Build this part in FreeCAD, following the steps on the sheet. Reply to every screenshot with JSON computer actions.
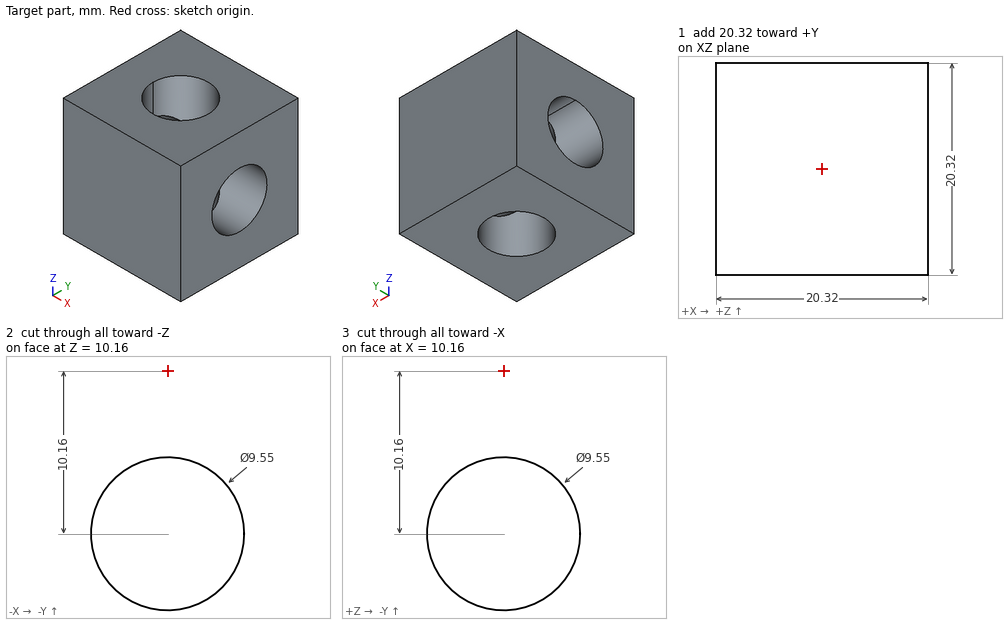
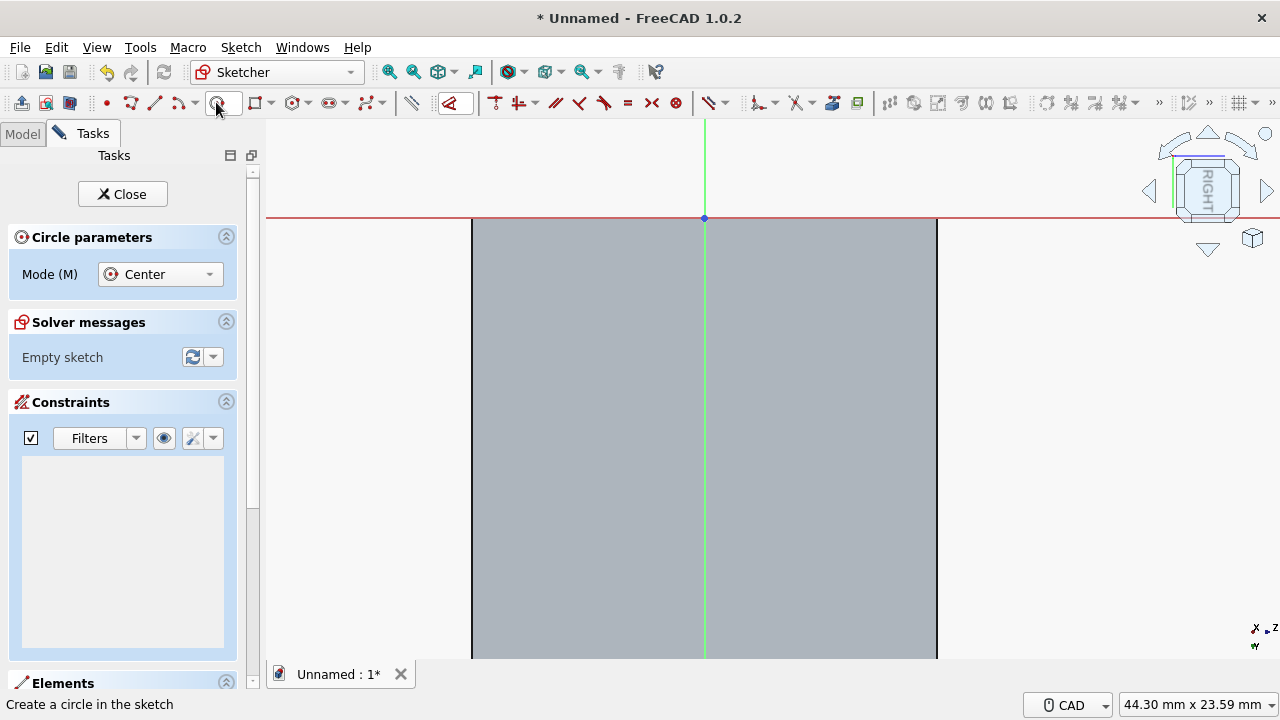
{"action": "left_click", "coordinate": [705, 451]}
{"action": "mouse_move", "coordinate": [782, 373]}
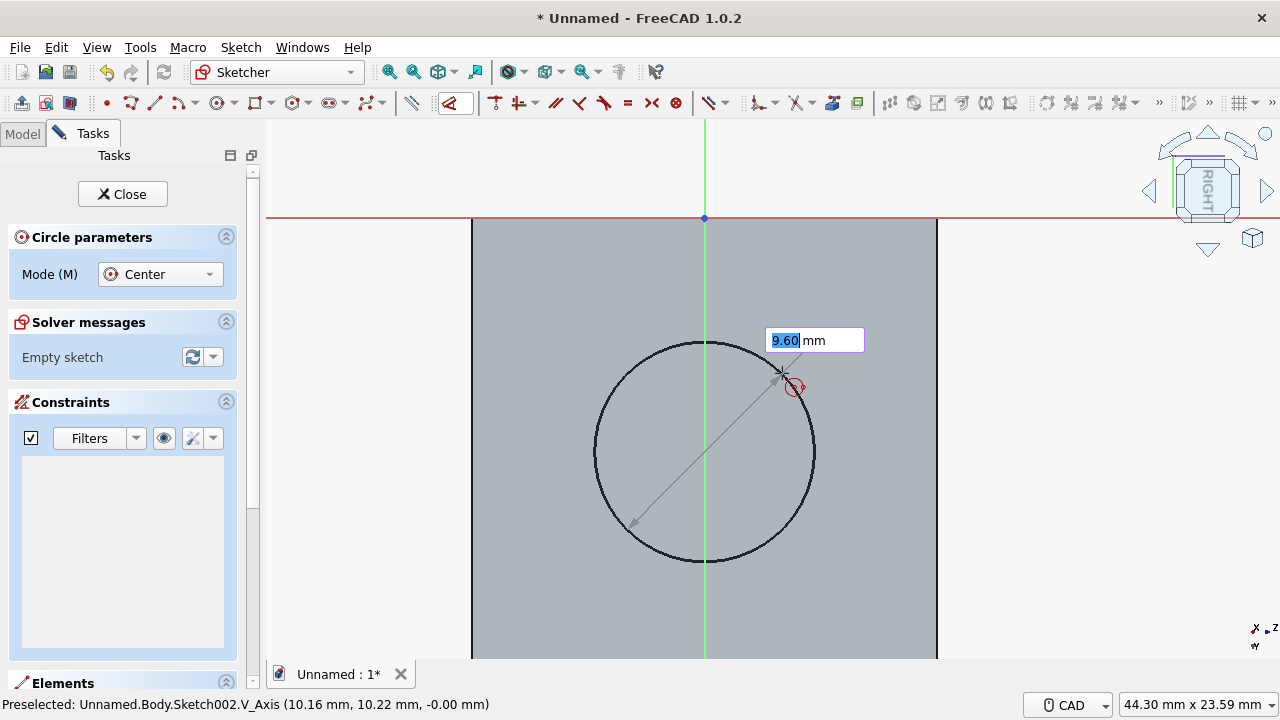
{"action": "type", "text": "9.55"}
{"action": "key", "text": "Return"}
{"action": "key", "text": "Escape"}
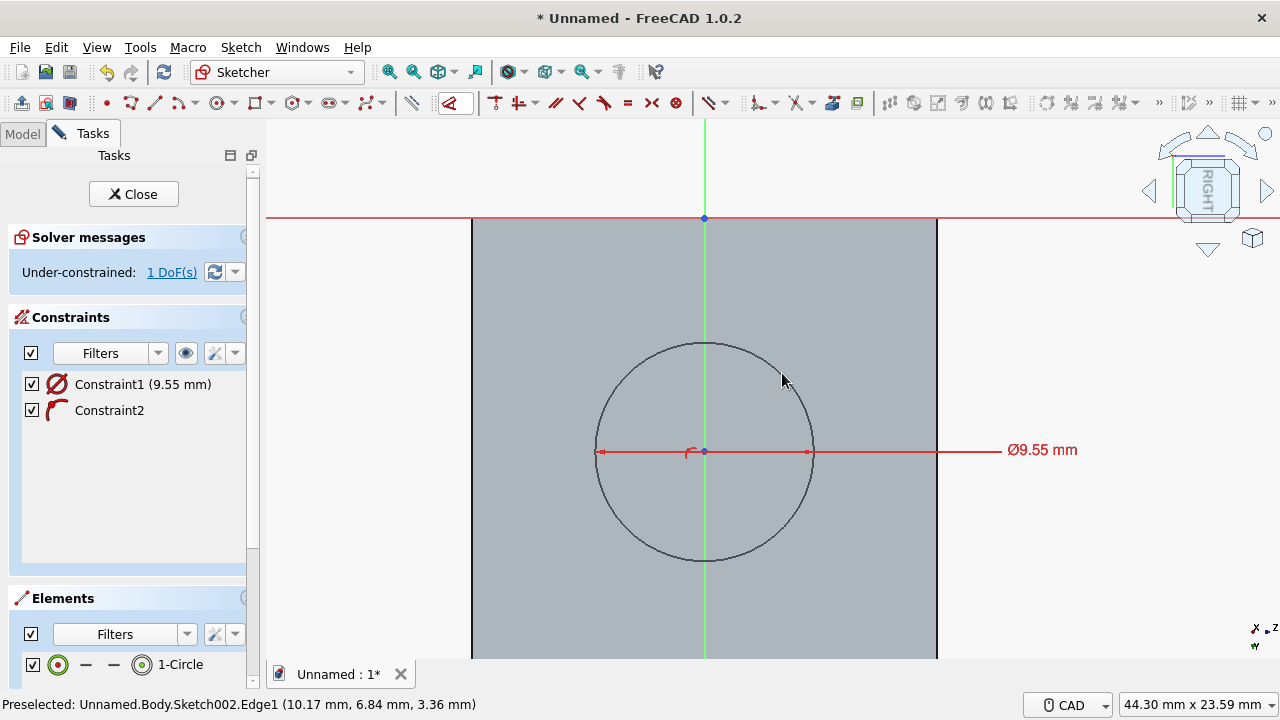
{"action": "left_click", "coordinate": [705, 452]}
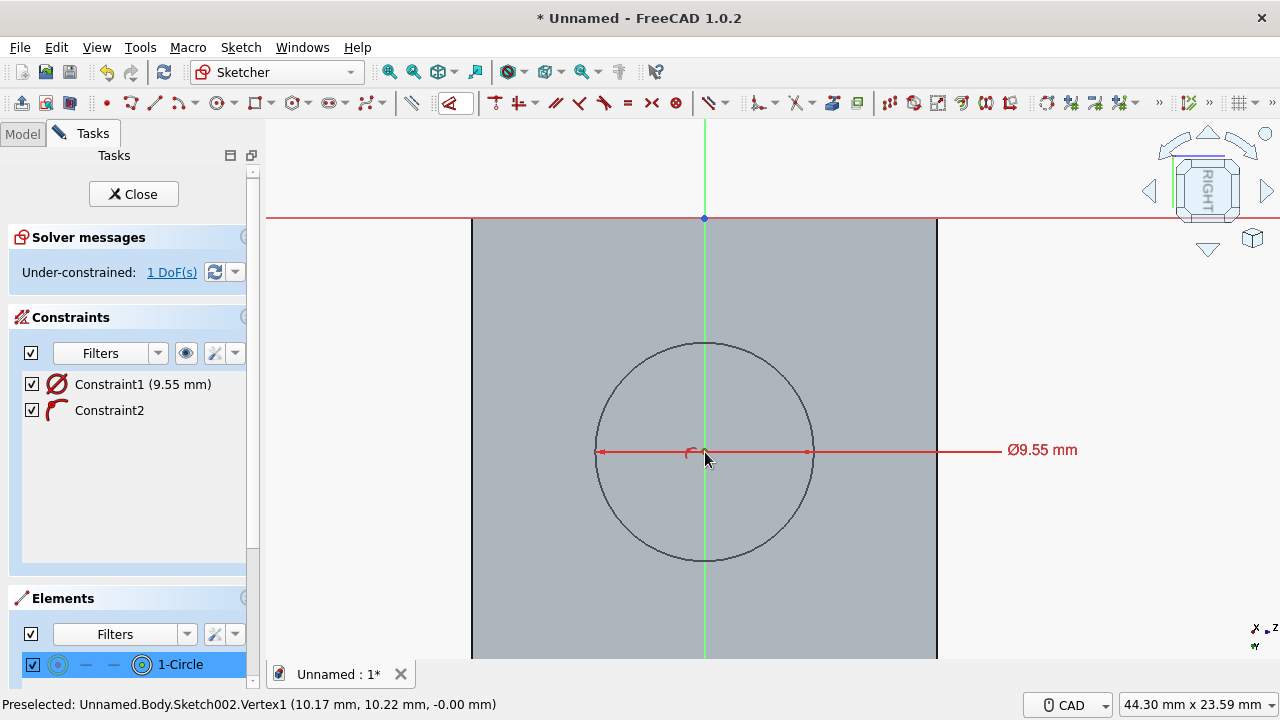
{"action": "key", "text": "i"}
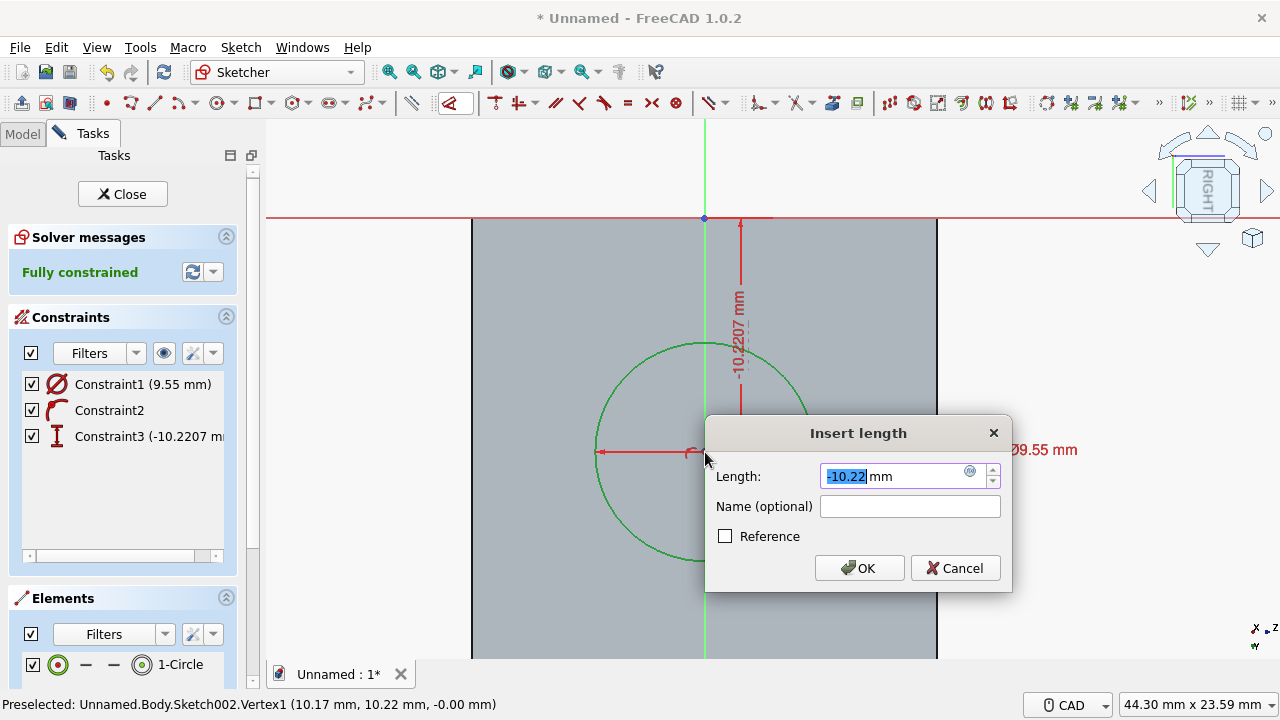
{"action": "type", "text": "-10.16"}
{"action": "key", "text": "Return"}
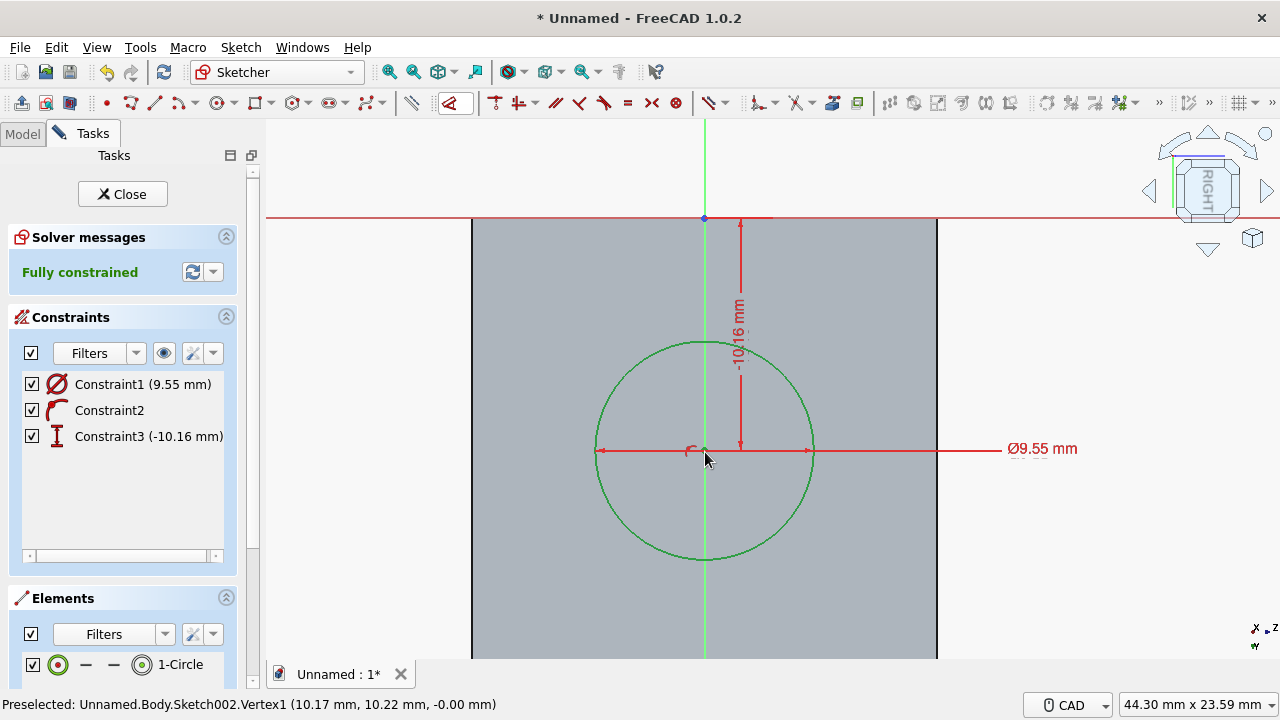
{"action": "left_click", "coordinate": [123, 194]}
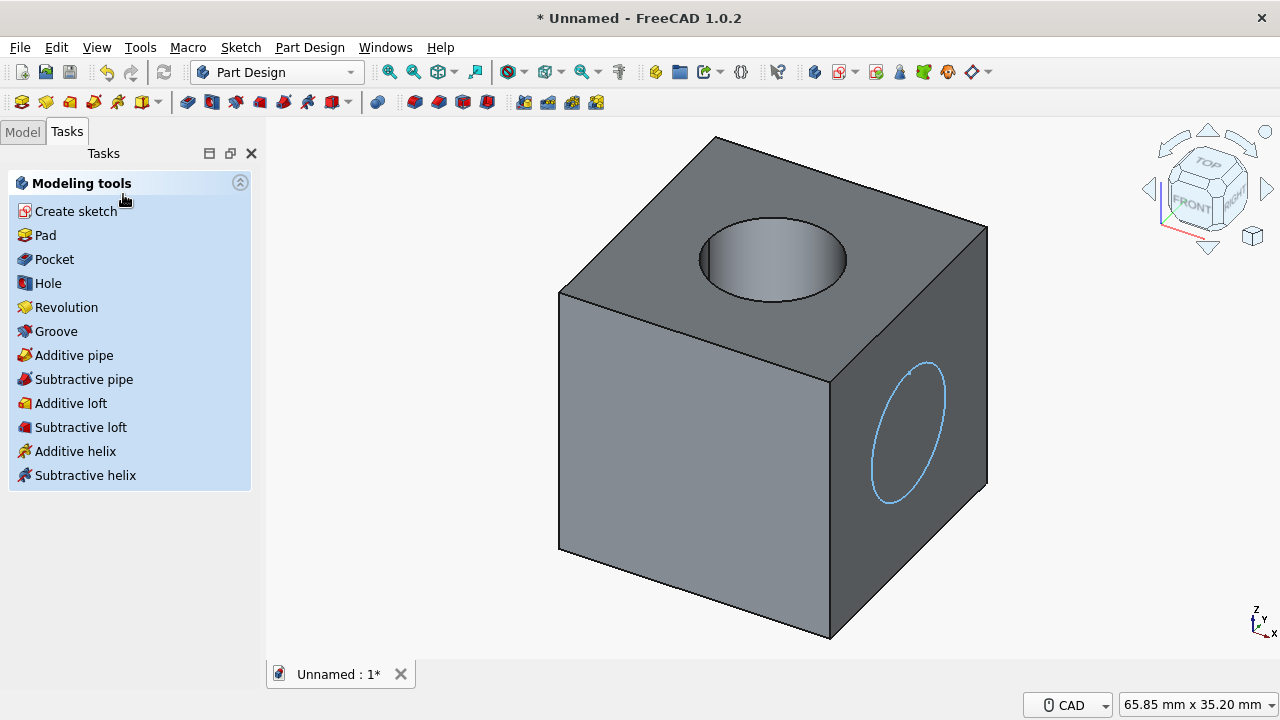
{"action": "left_click", "coordinate": [188, 102]}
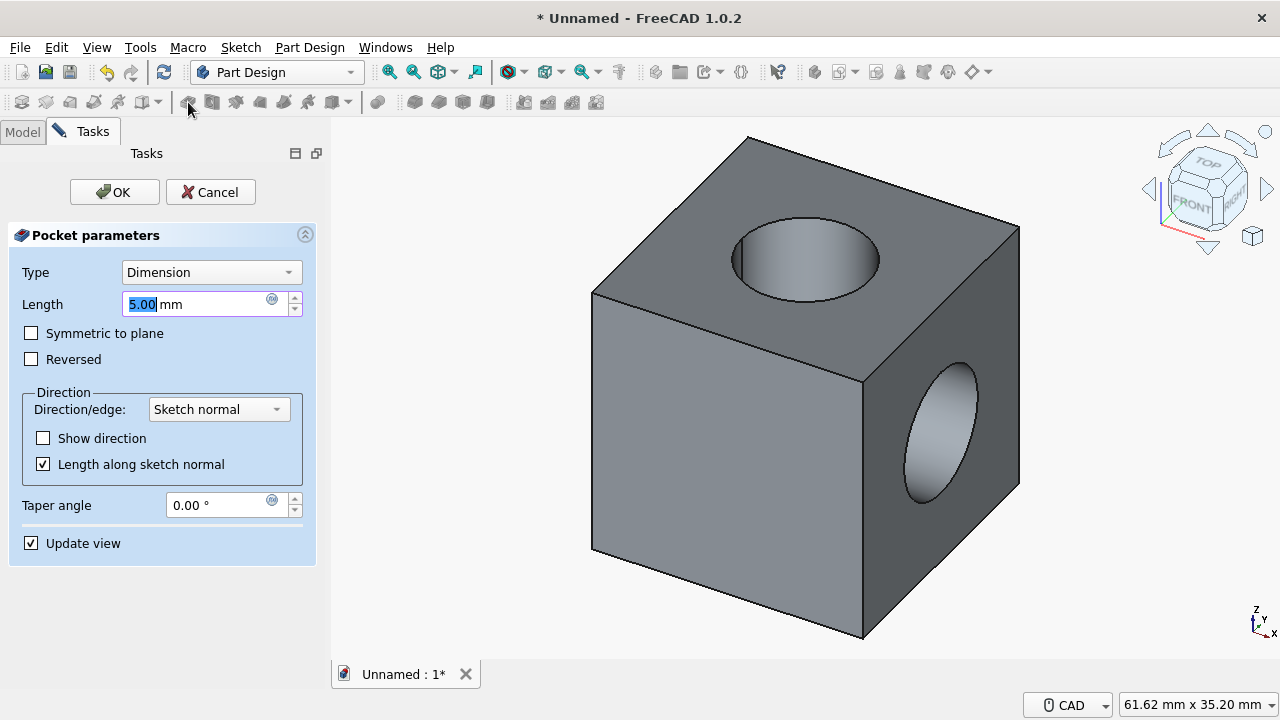
{"action": "left_click", "coordinate": [212, 272]}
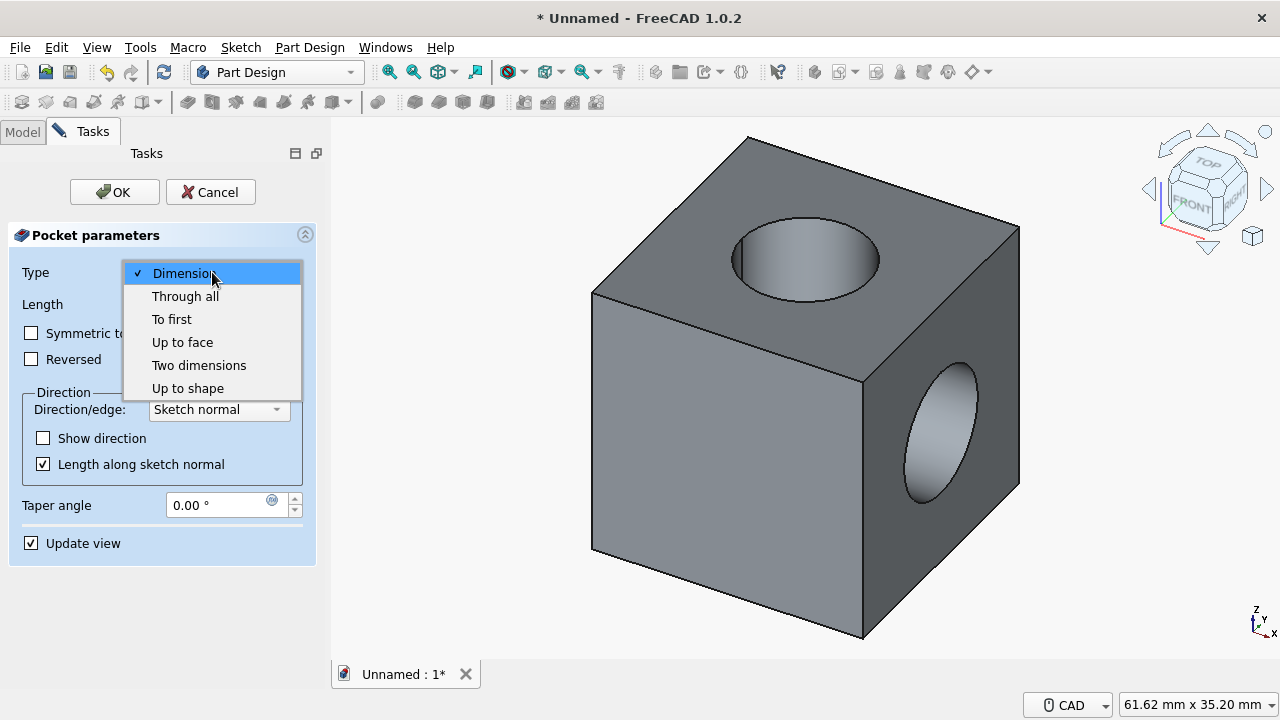
{"action": "left_click", "coordinate": [212, 296]}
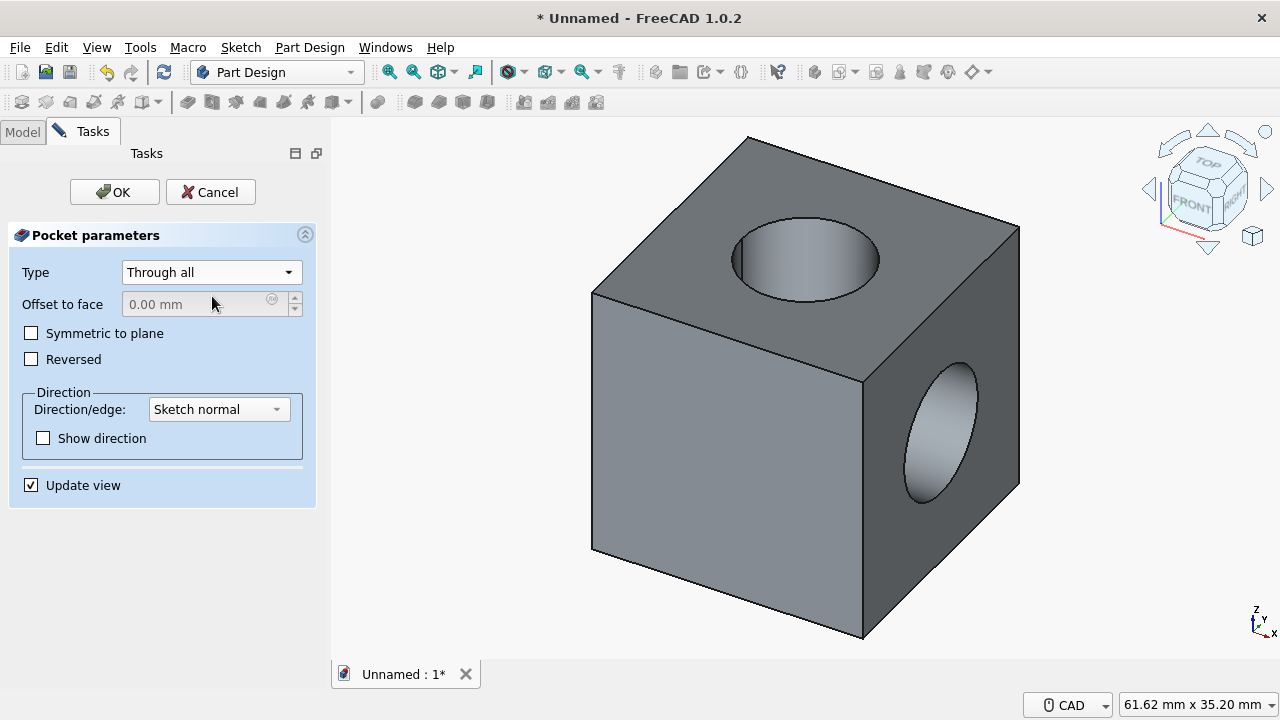
{"action": "left_click", "coordinate": [115, 192]}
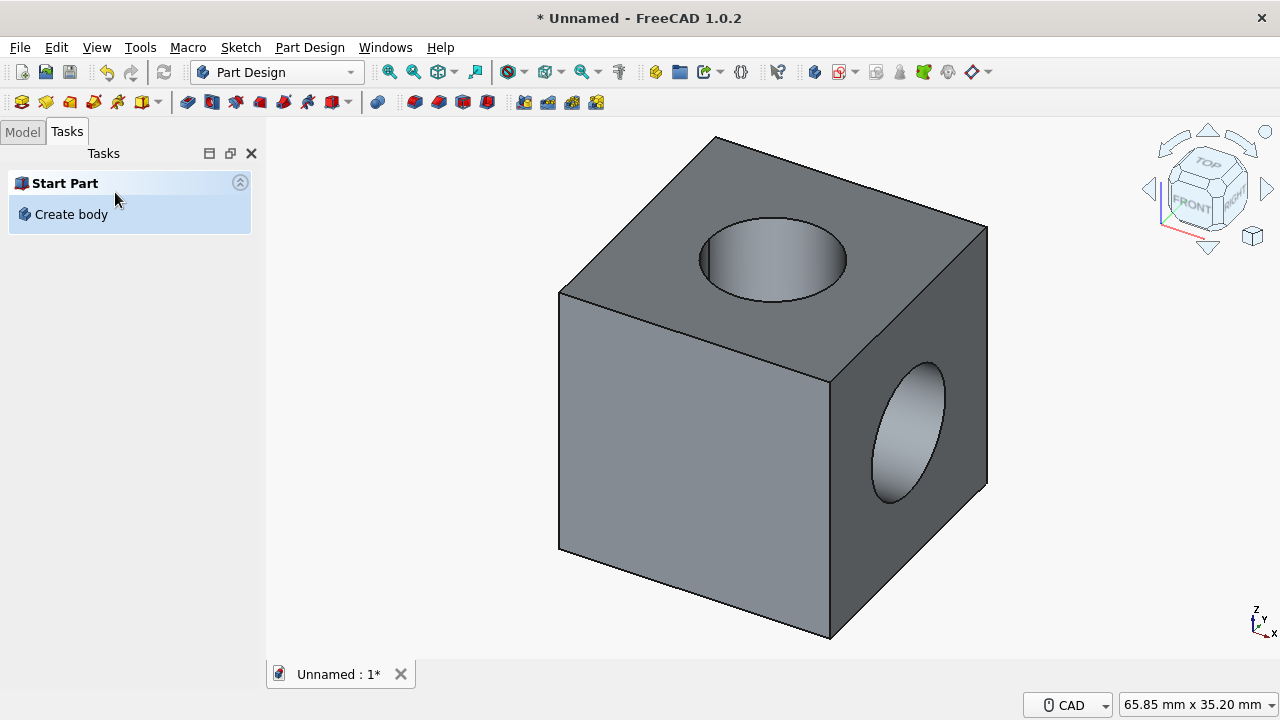
{"action": "key", "text": "0"}